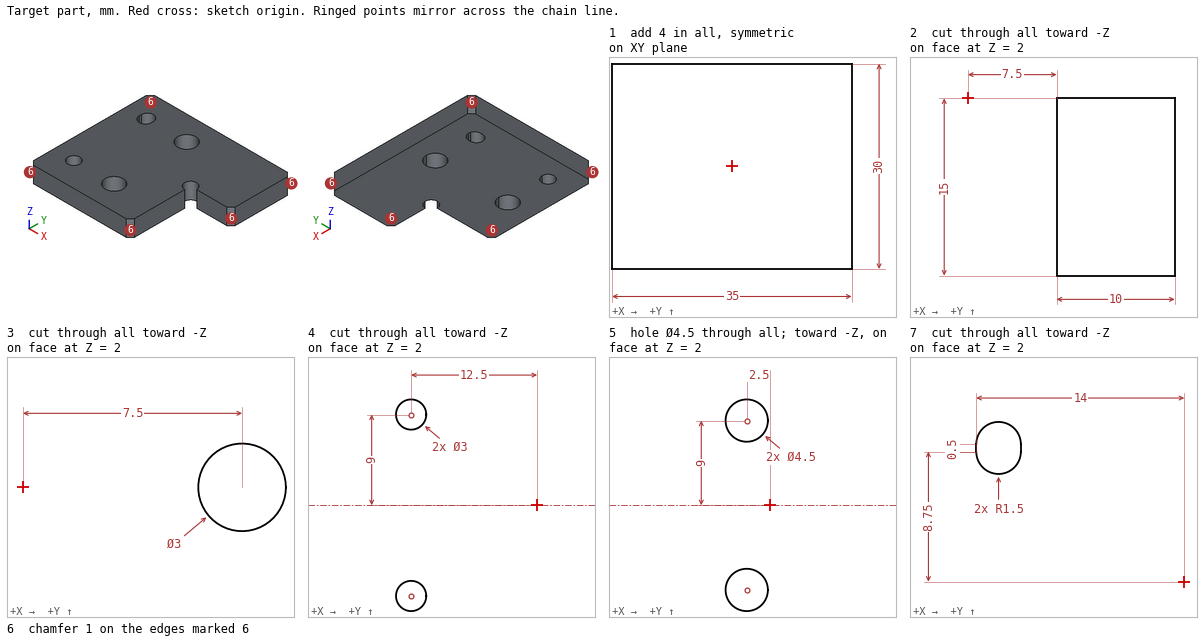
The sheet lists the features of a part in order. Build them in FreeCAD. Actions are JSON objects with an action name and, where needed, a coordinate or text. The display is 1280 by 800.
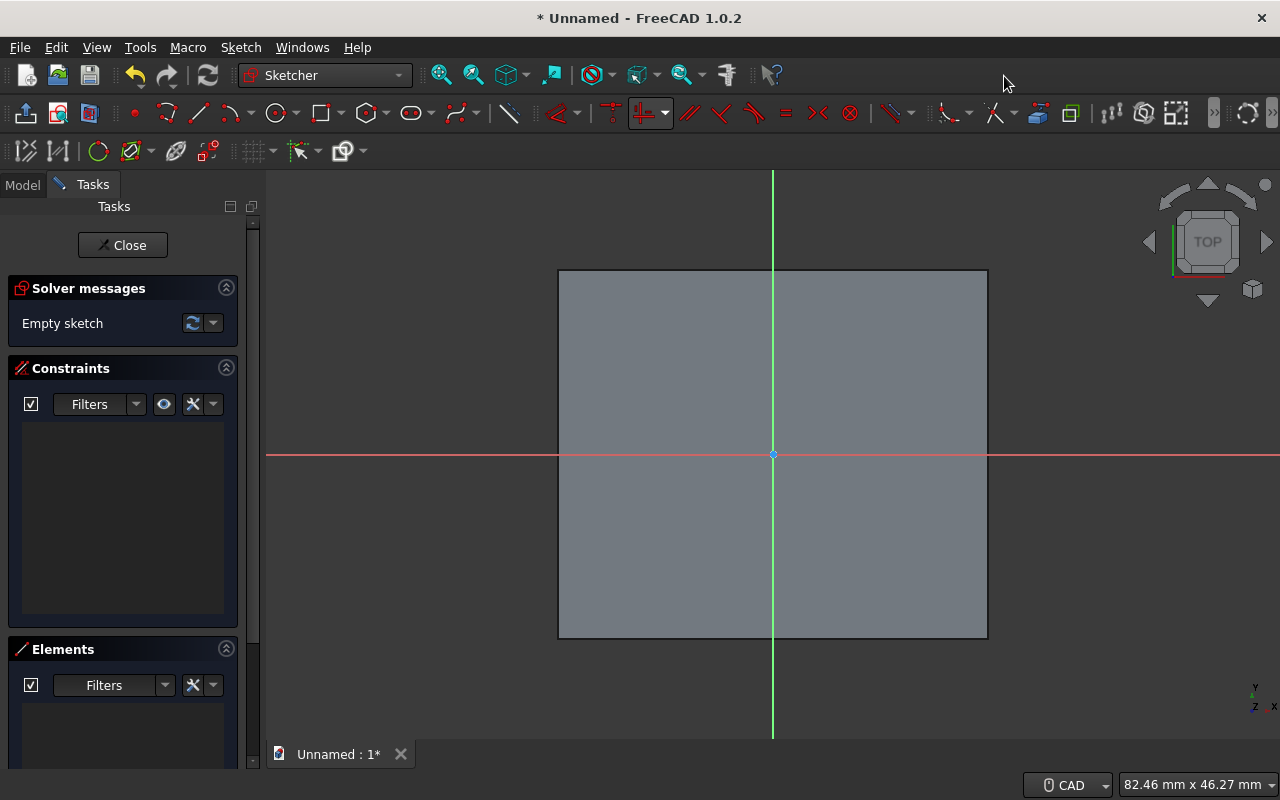
{"action": "scroll", "coordinate": [1095, 659], "scroll_direction": "up", "scroll_amount": 3}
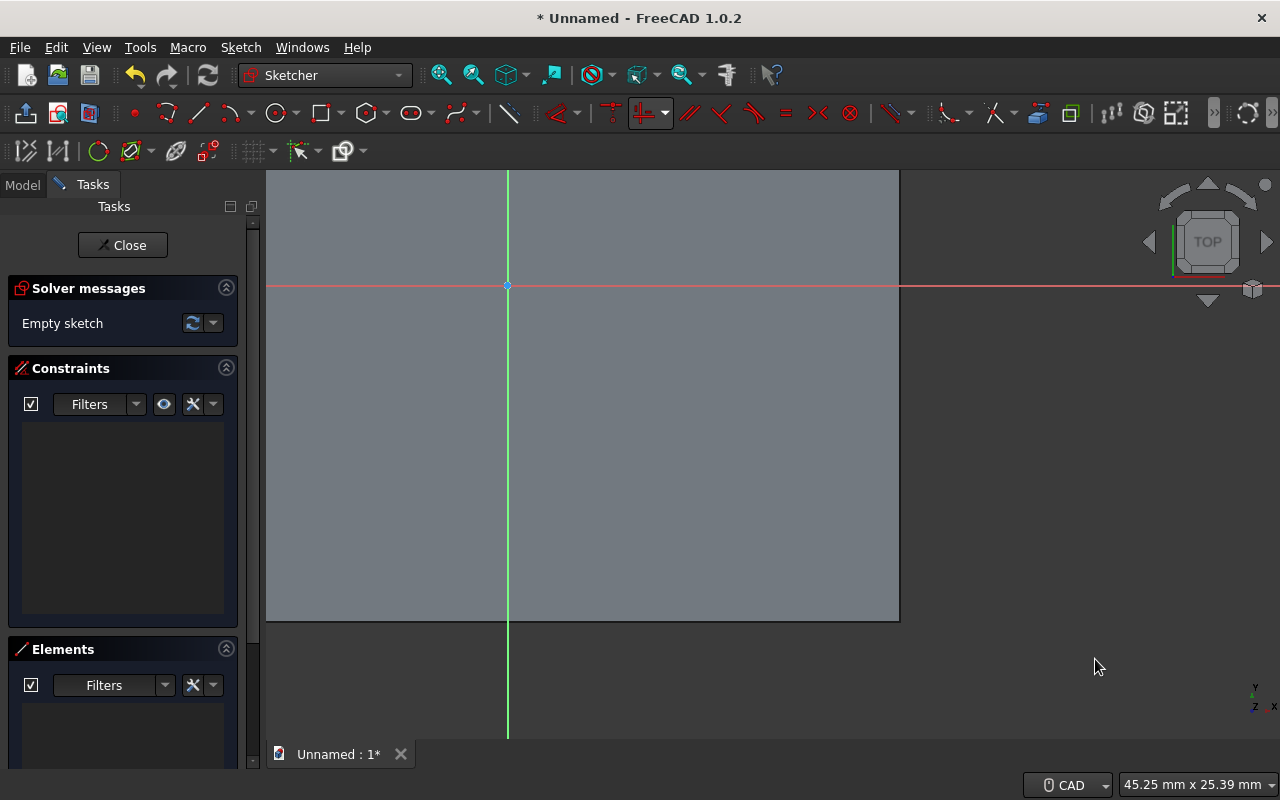
{"action": "left_click", "coordinate": [322, 114]}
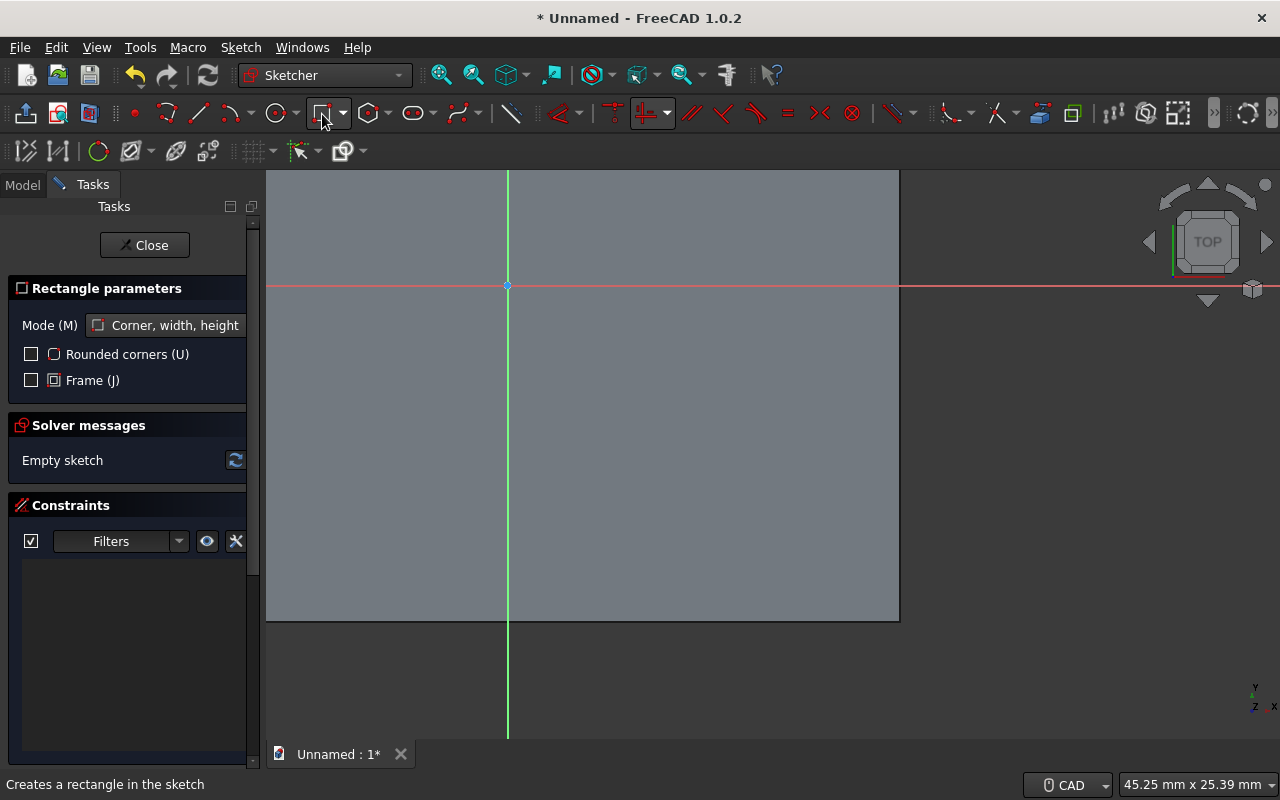
{"action": "left_click", "coordinate": [676, 286]}
{"action": "left_click", "coordinate": [900, 622]}
{"action": "key", "text": "Escape"}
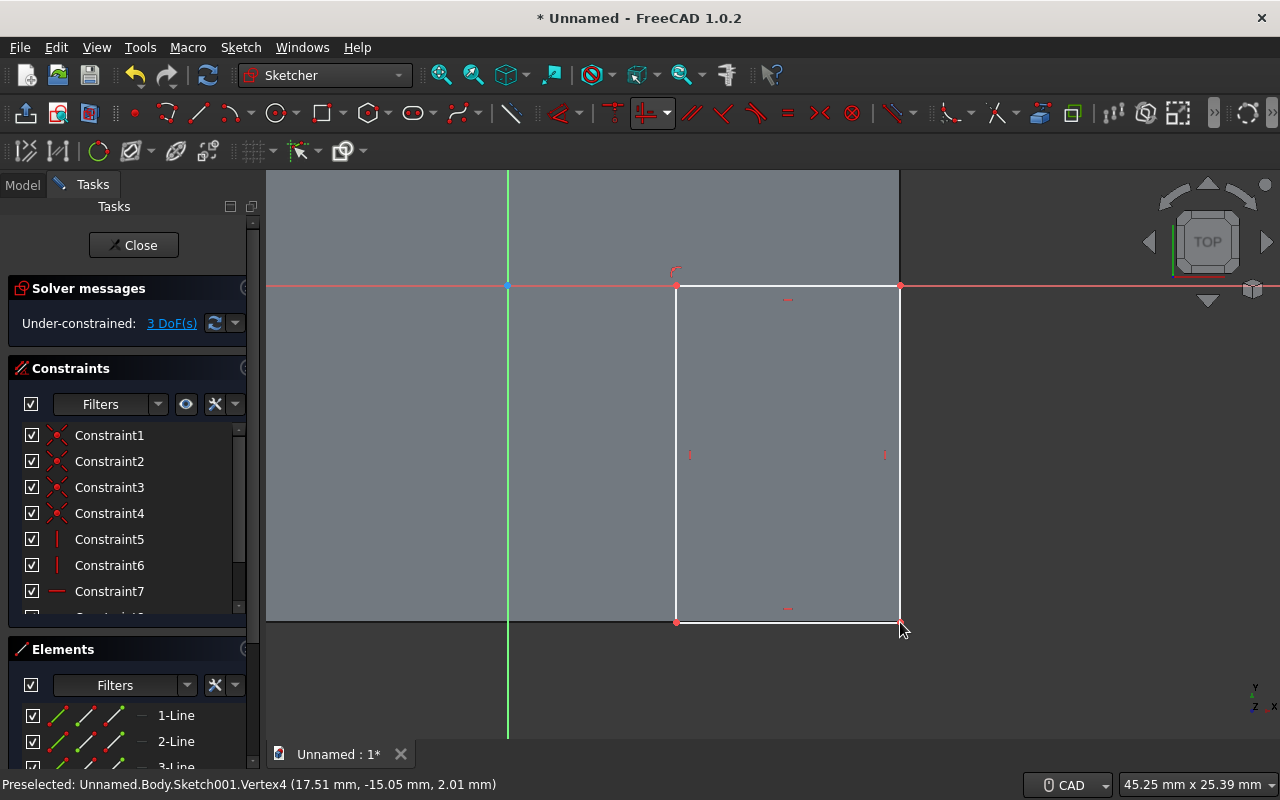
{"action": "left_click", "coordinate": [558, 114]}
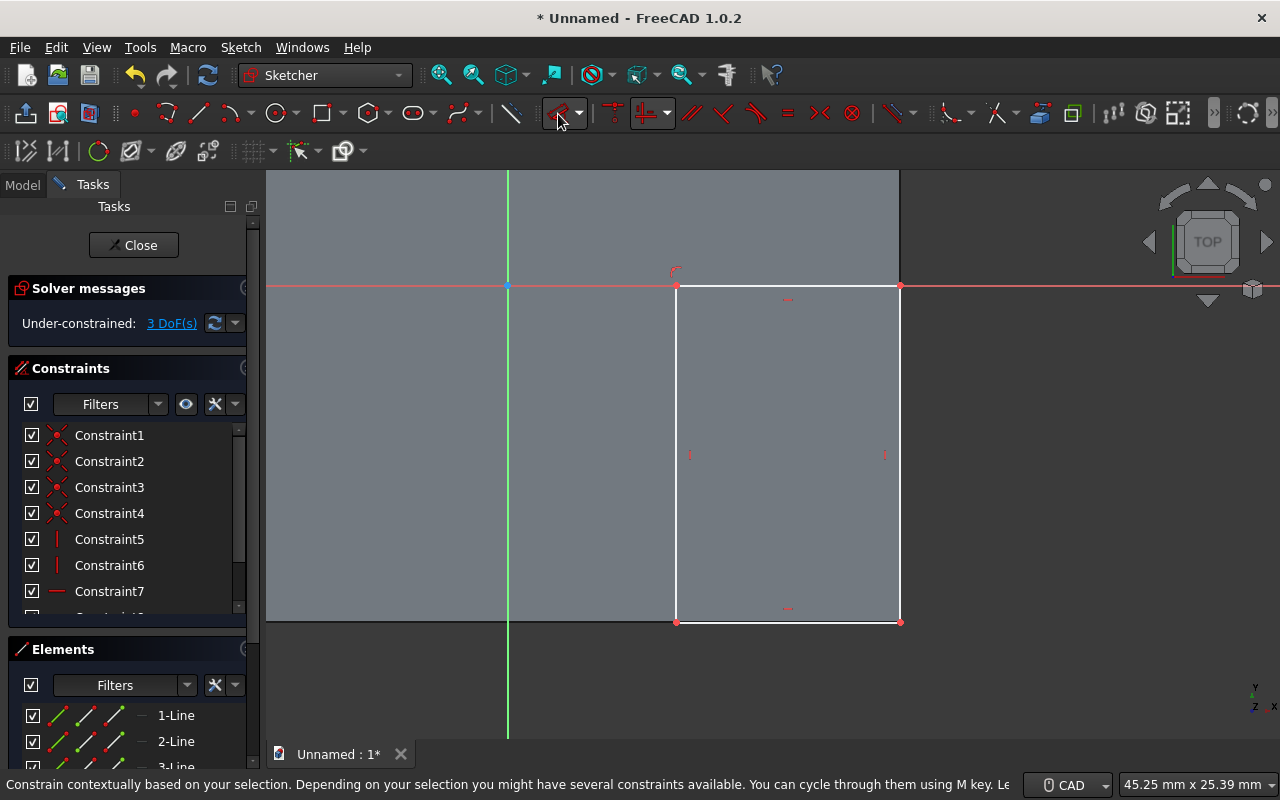
{"action": "left_click", "coordinate": [676, 387]}
{"action": "left_click", "coordinate": [642, 454]}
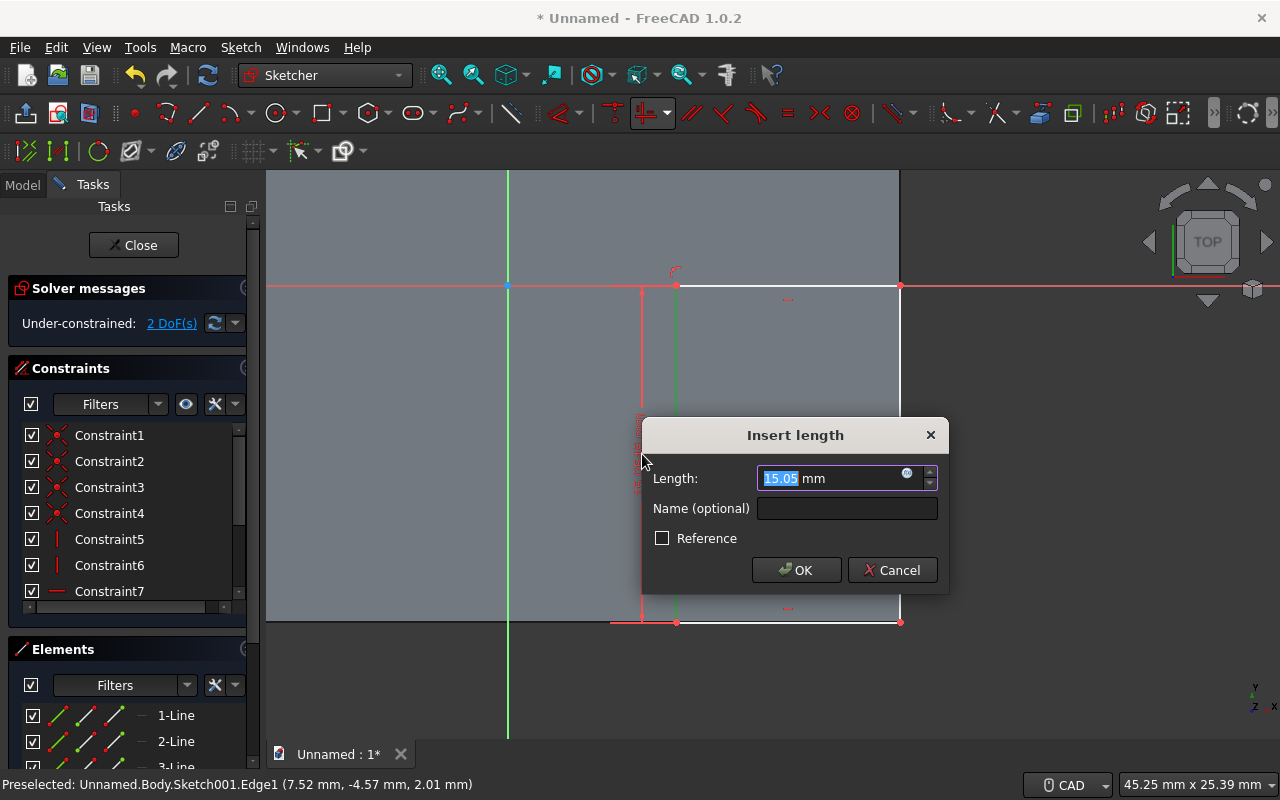
{"action": "type", "text": "15"}
{"action": "key", "text": "Return"}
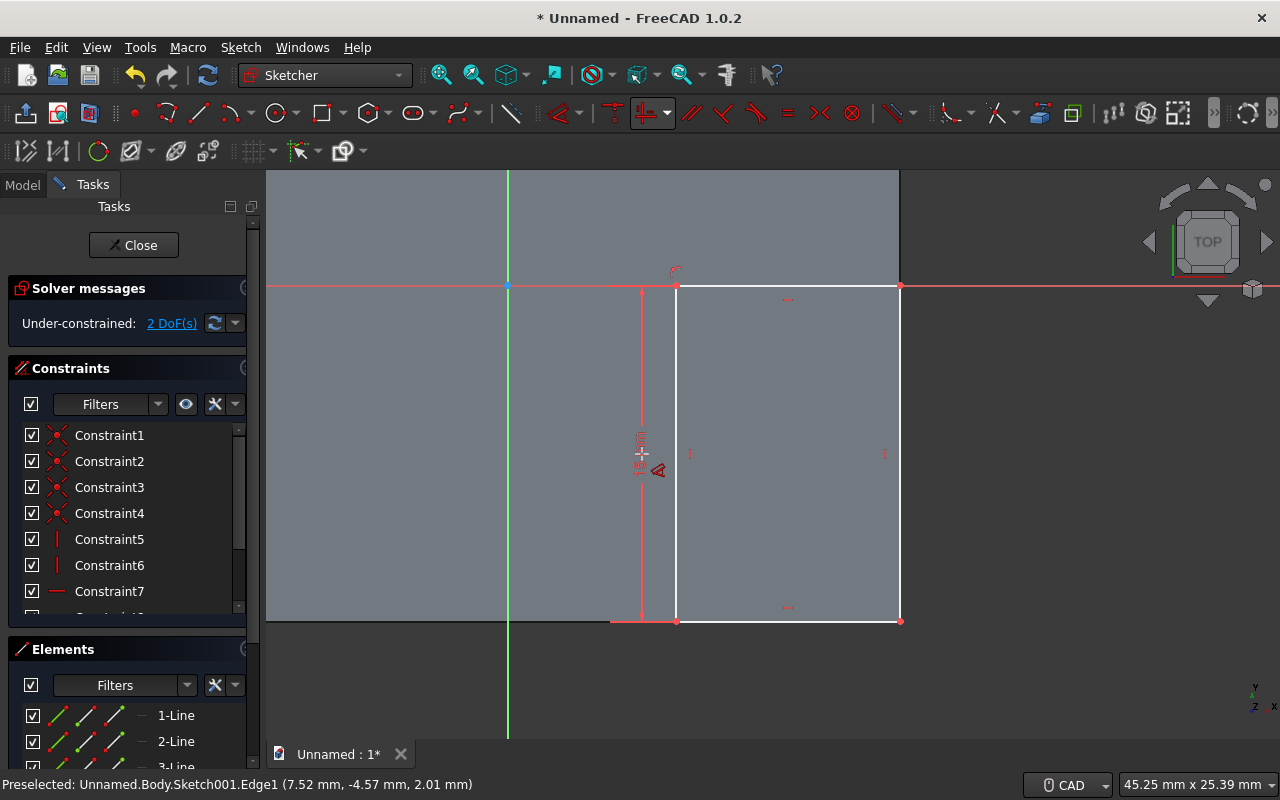
{"action": "left_click", "coordinate": [743, 622]}
{"action": "left_click", "coordinate": [788, 656]}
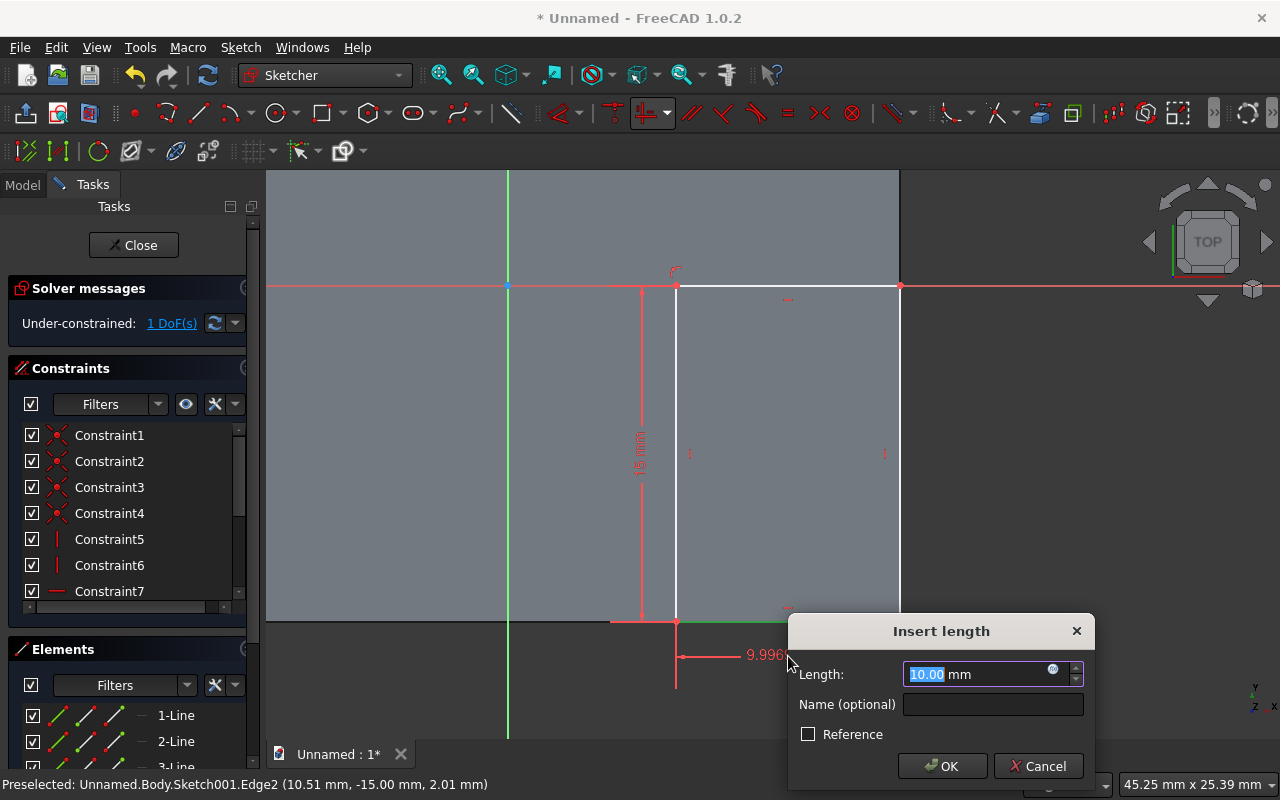
{"action": "type", "text": "10"}
{"action": "key", "text": "Return"}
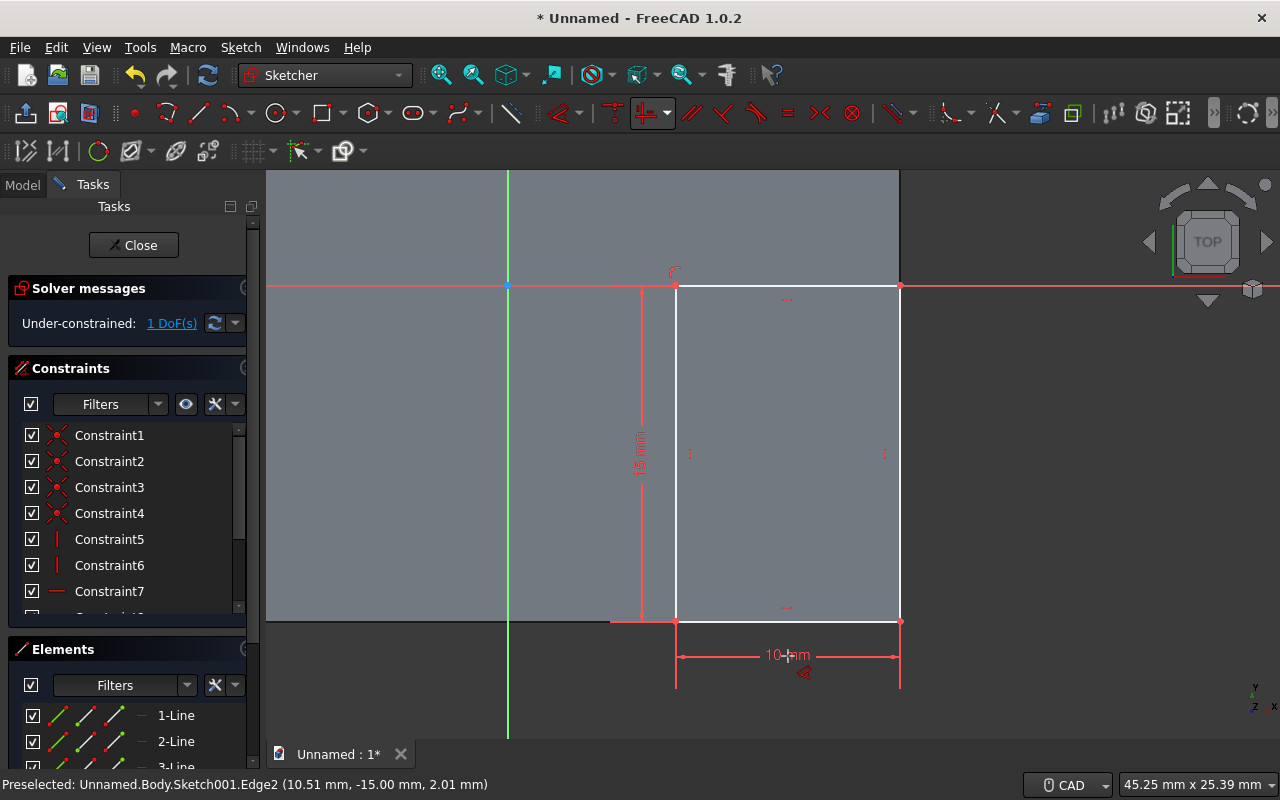
{"action": "left_click", "coordinate": [676, 286]}
{"action": "left_click", "coordinate": [592, 252]}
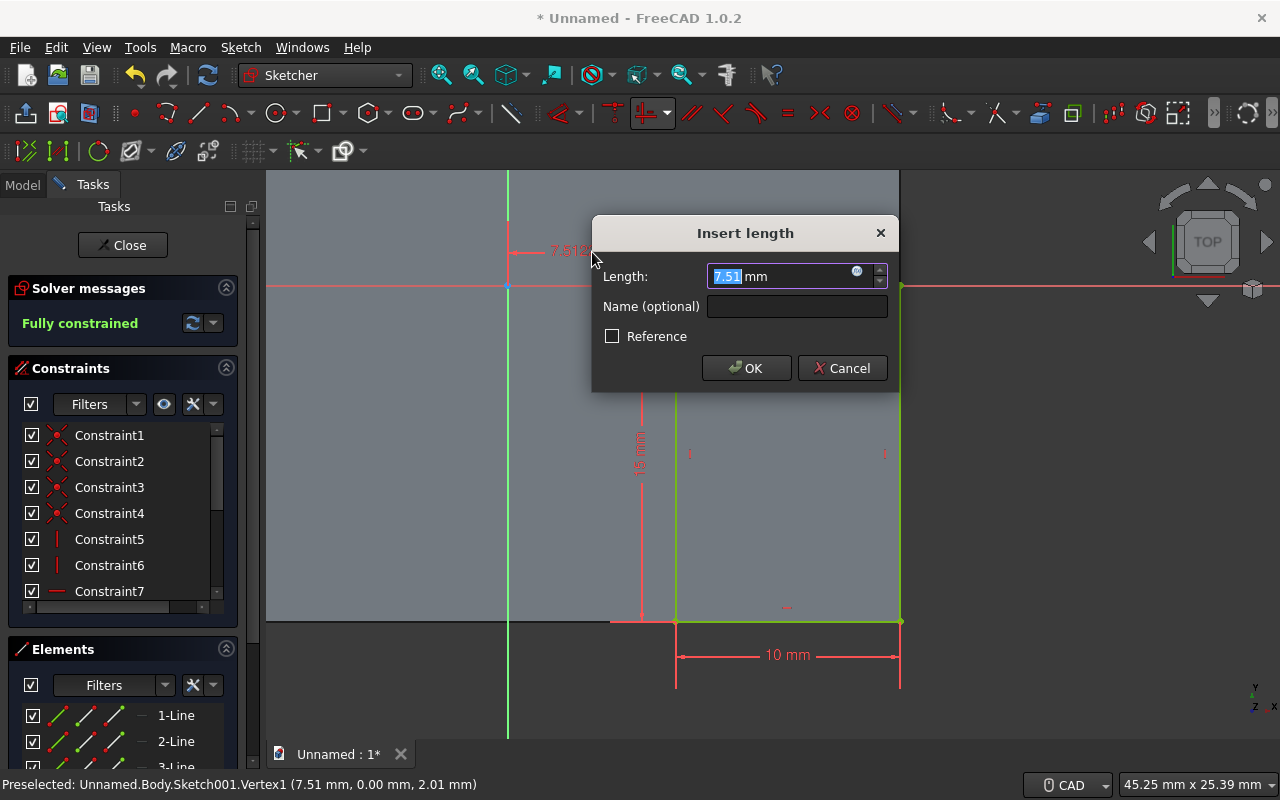
{"action": "type", "text": "7.5"}
{"action": "key", "text": "Return"}
{"action": "key", "text": "Escape"}